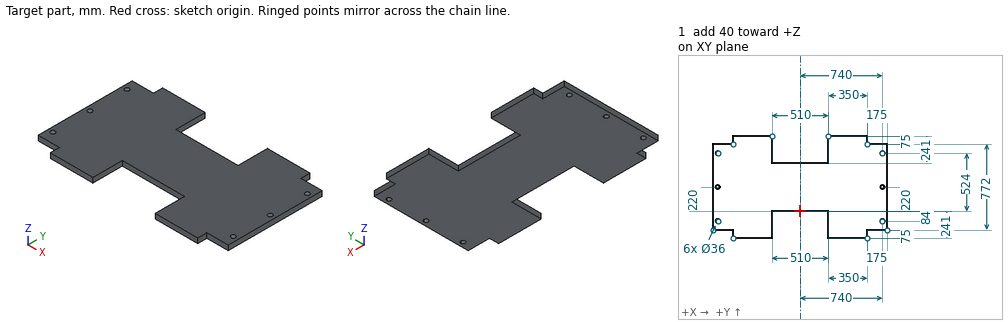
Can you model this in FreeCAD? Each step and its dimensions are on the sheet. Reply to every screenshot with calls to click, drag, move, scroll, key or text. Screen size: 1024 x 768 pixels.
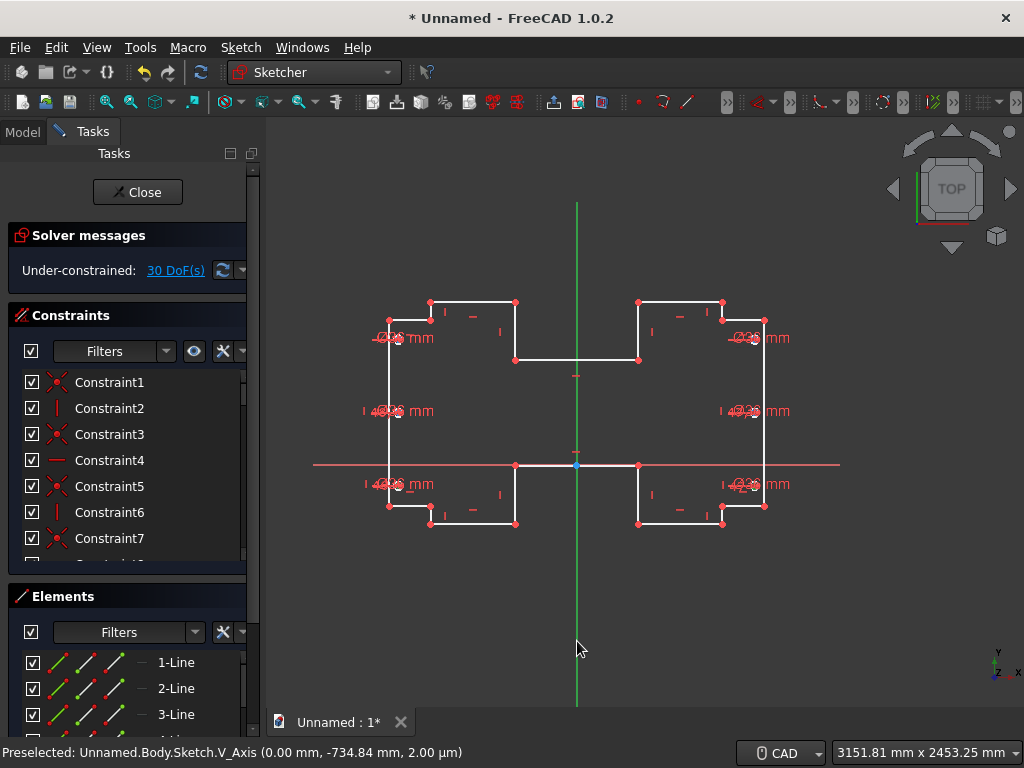
key(s)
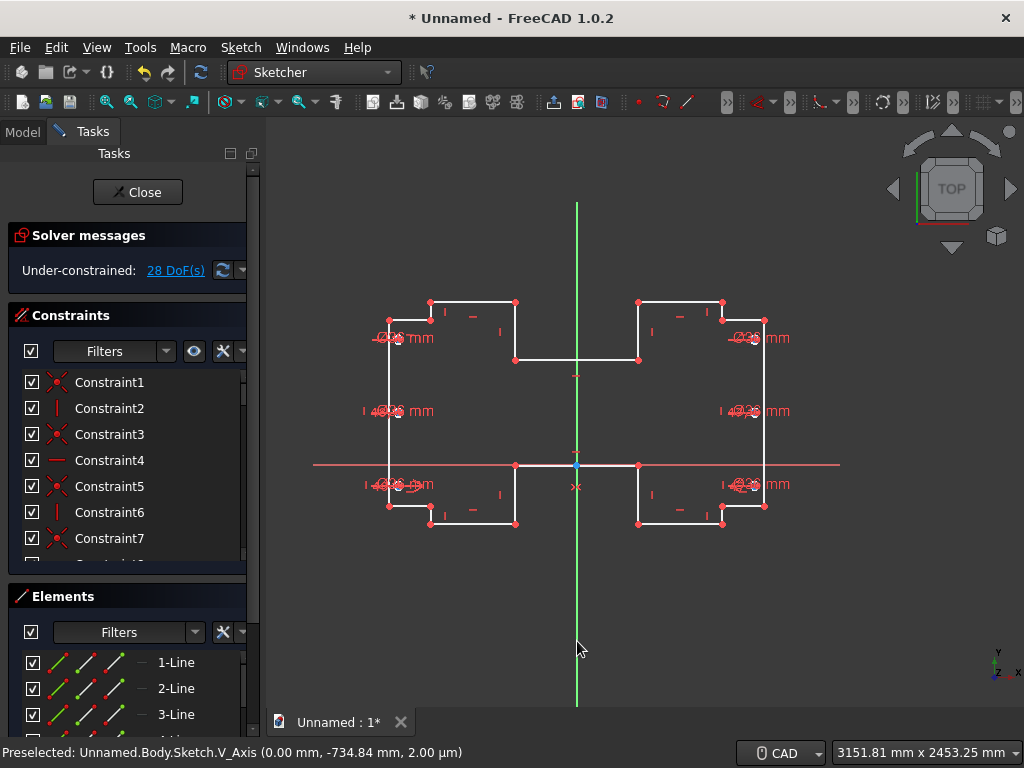
click(755, 340)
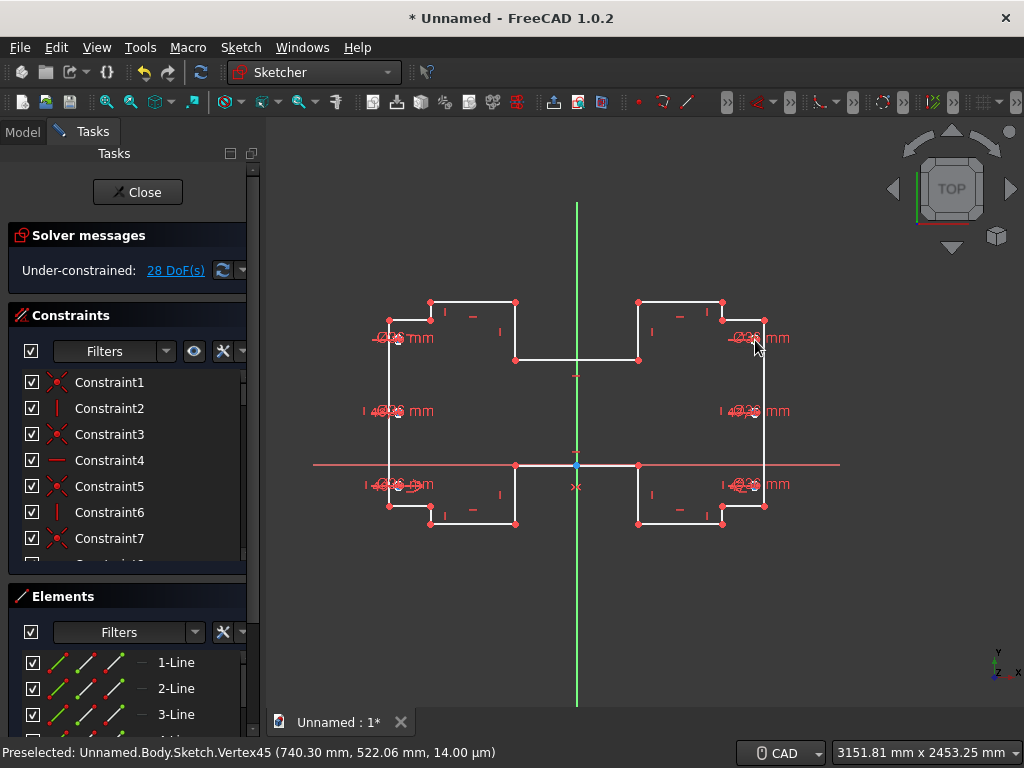
click(399, 340)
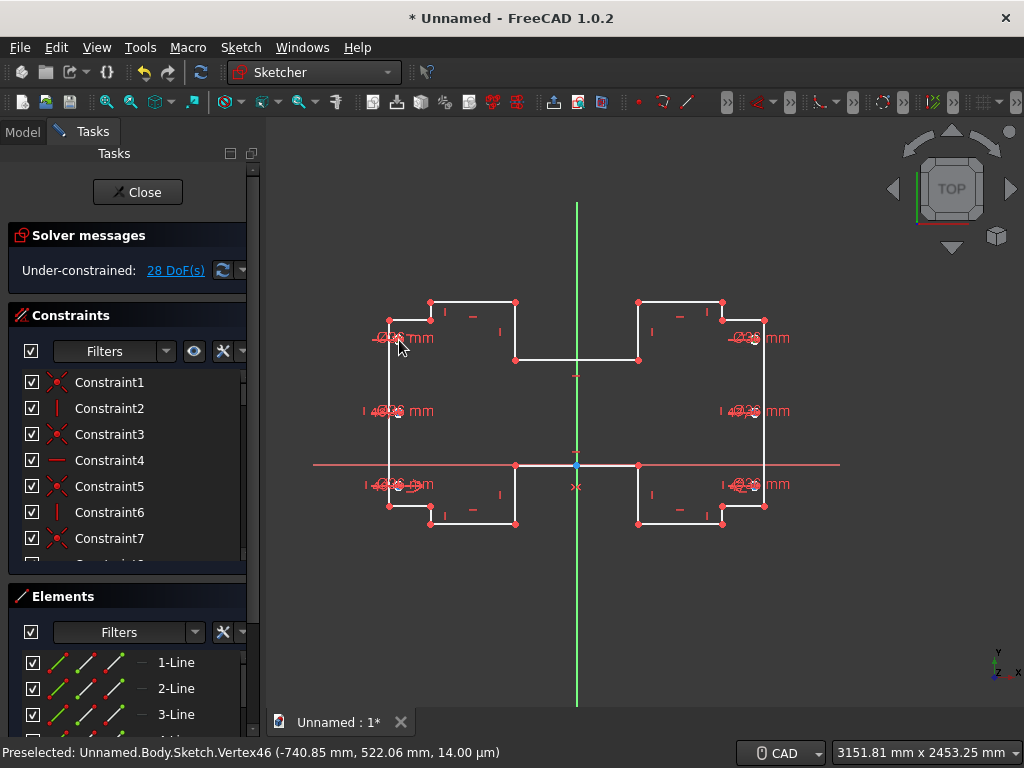
click(577, 641)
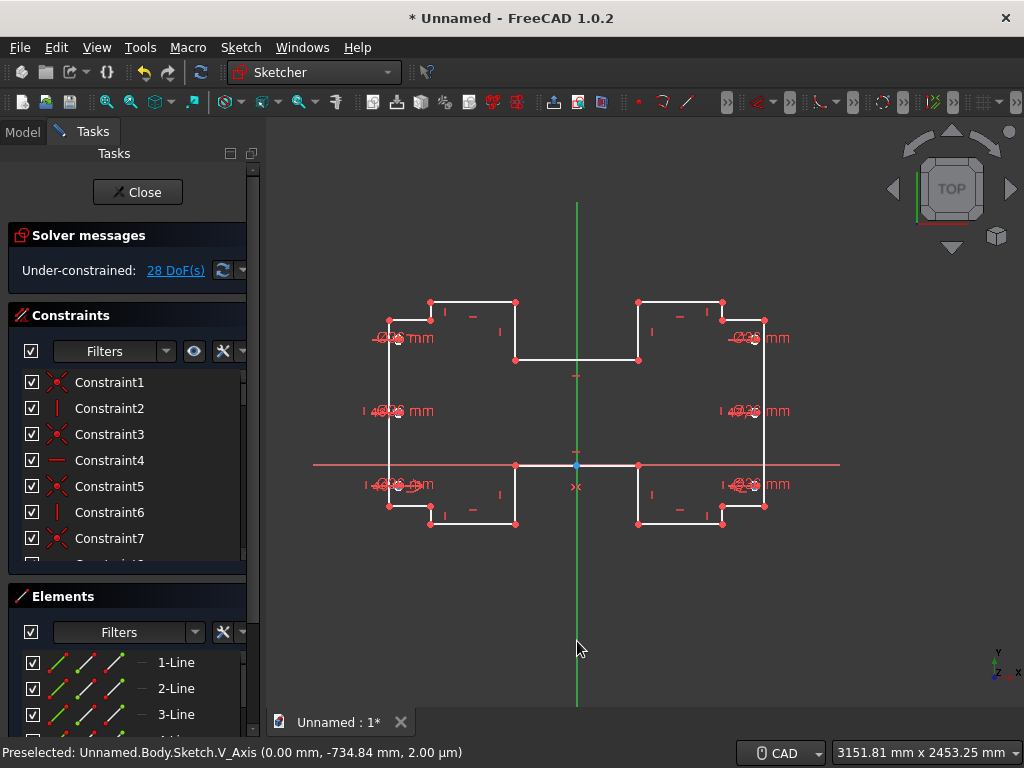
key(s)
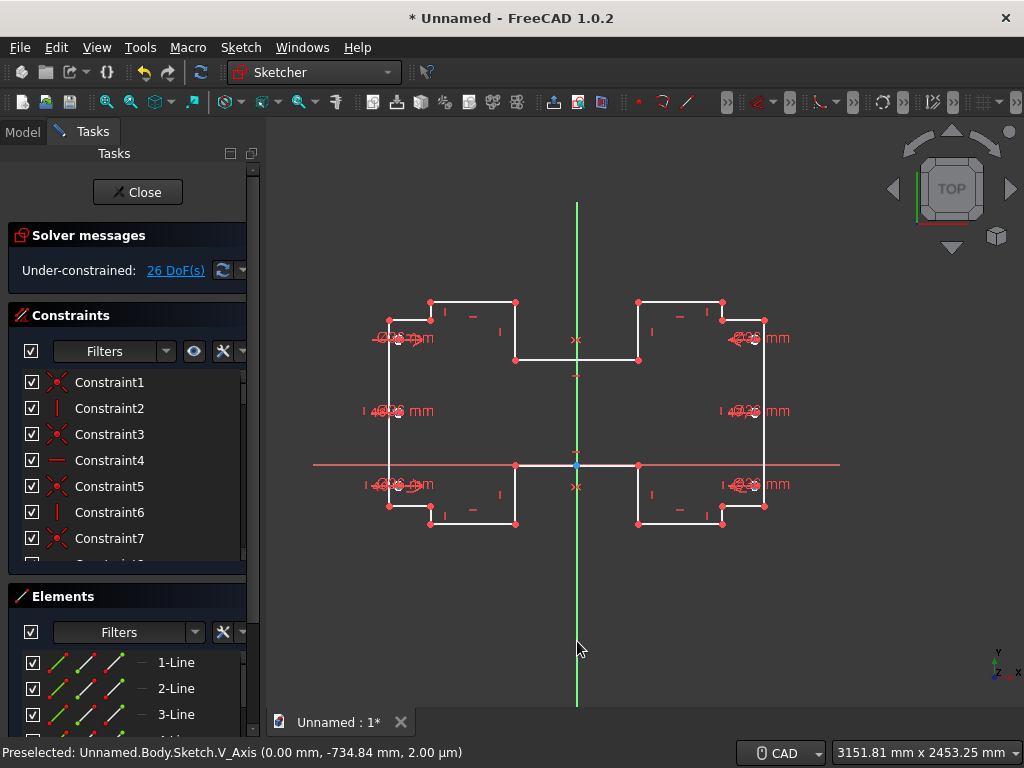
click(638, 302)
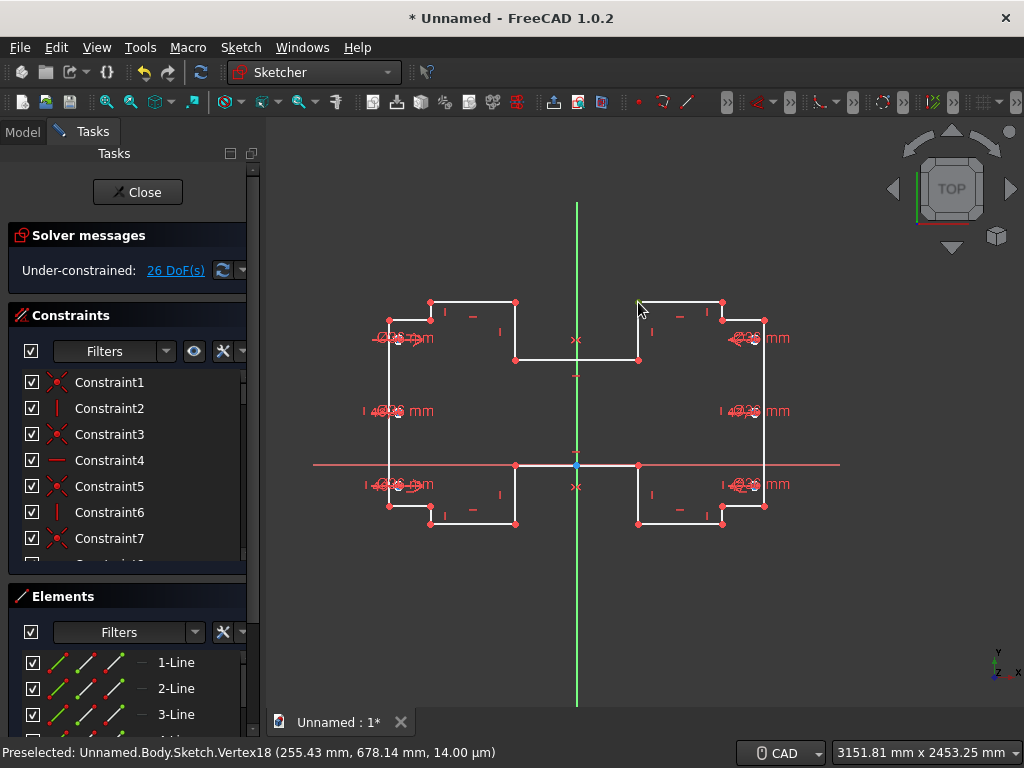
click(515, 302)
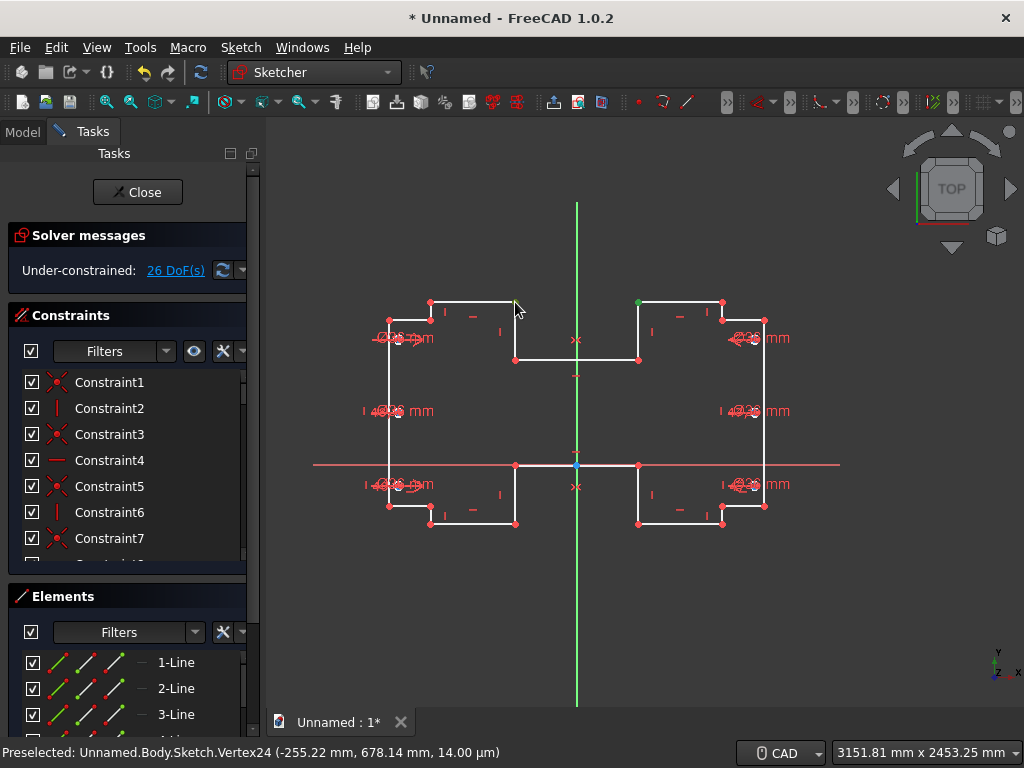
click(577, 641)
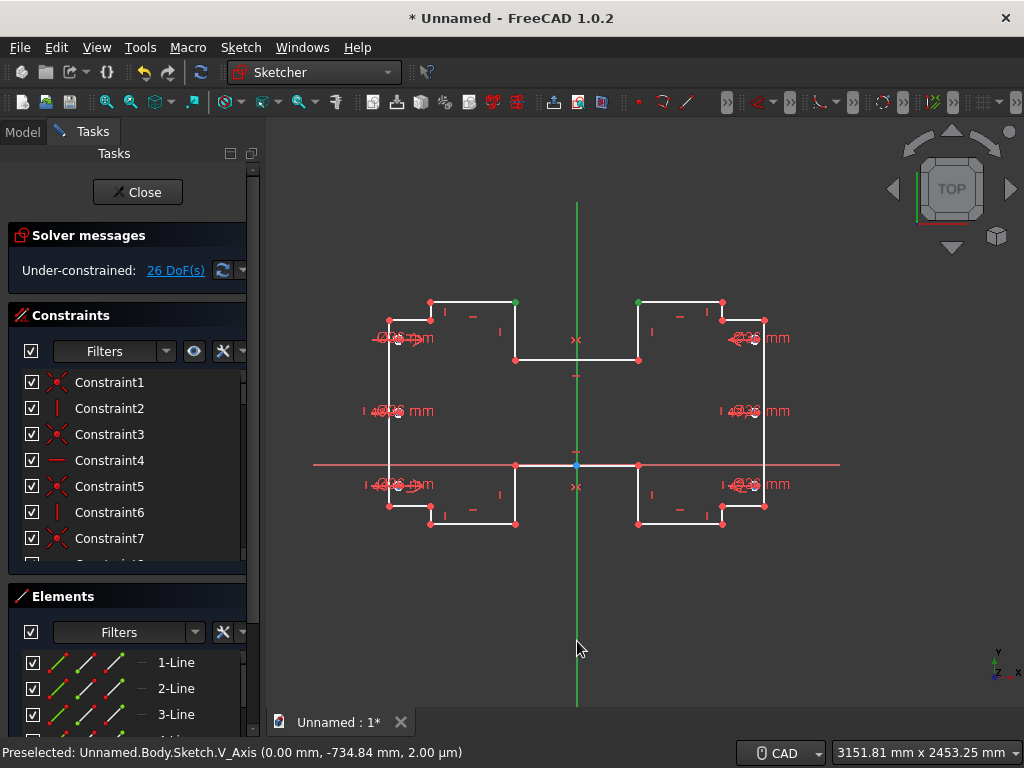
key(s)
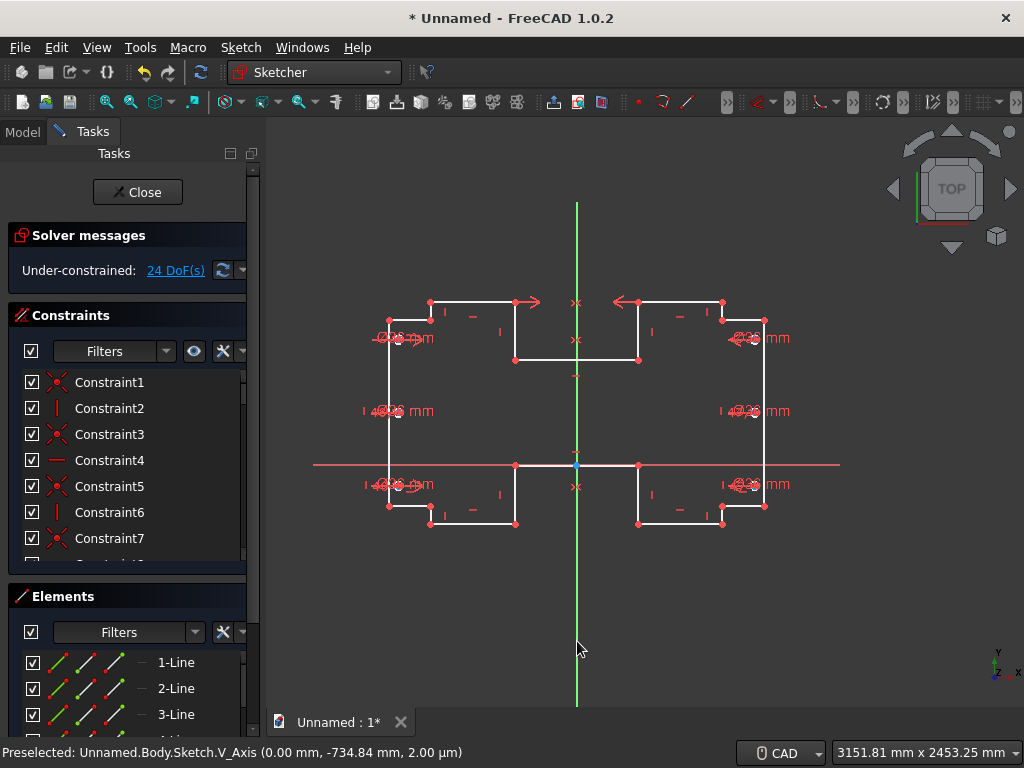
click(722, 320)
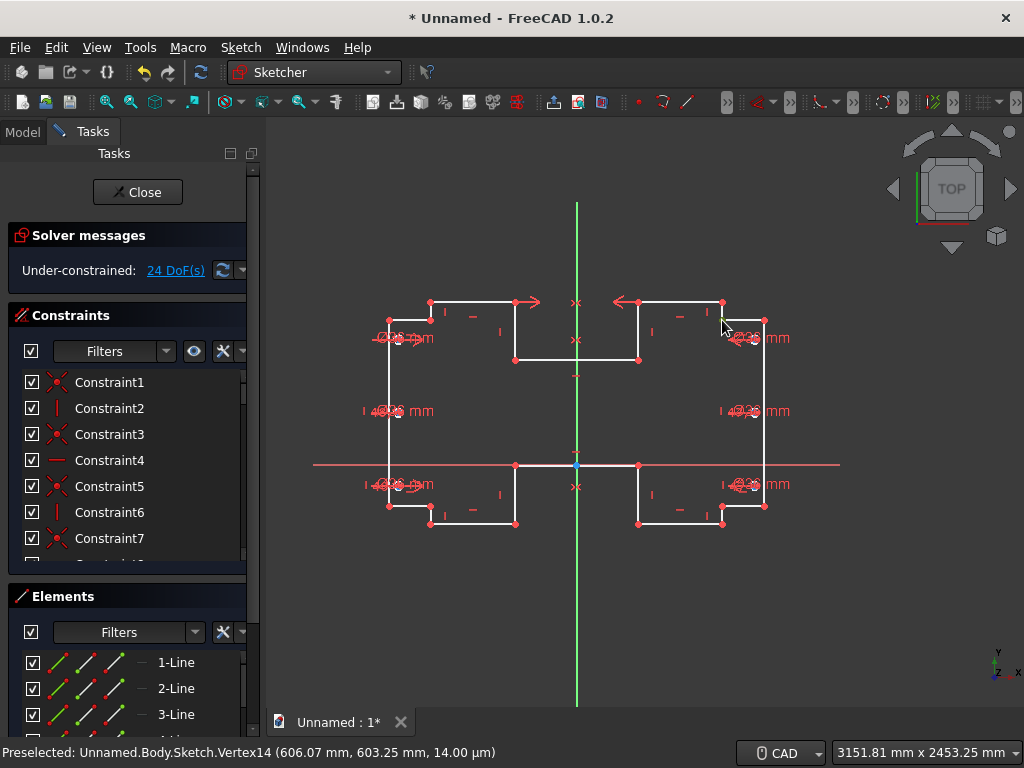
click(431, 320)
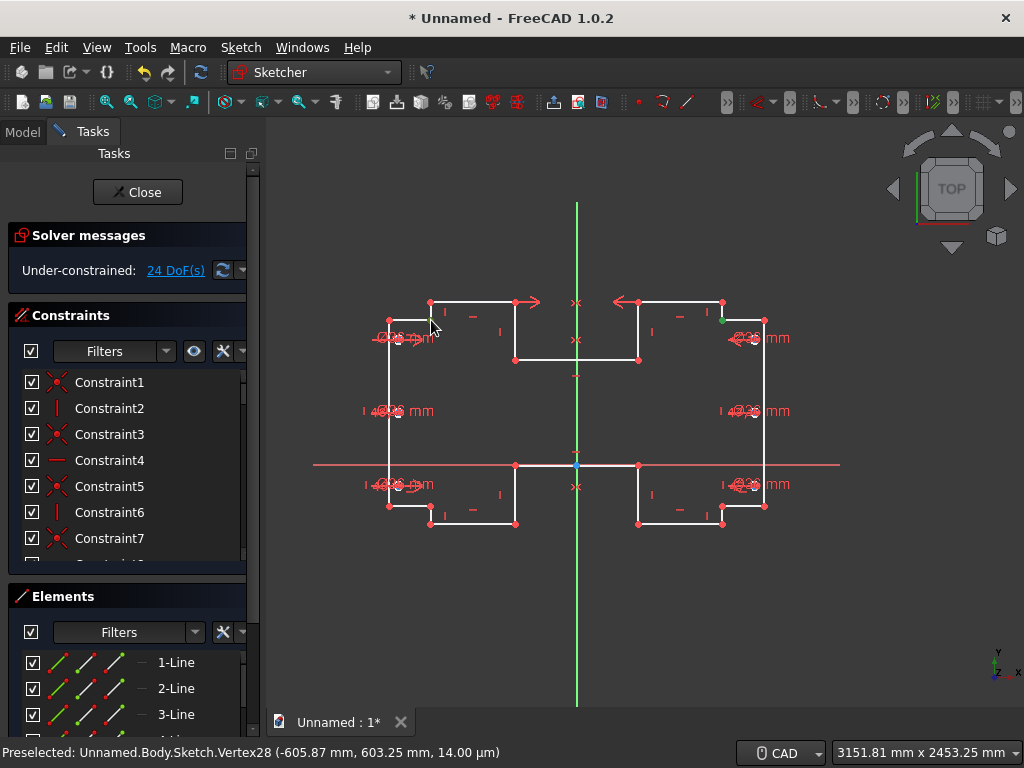
click(577, 641)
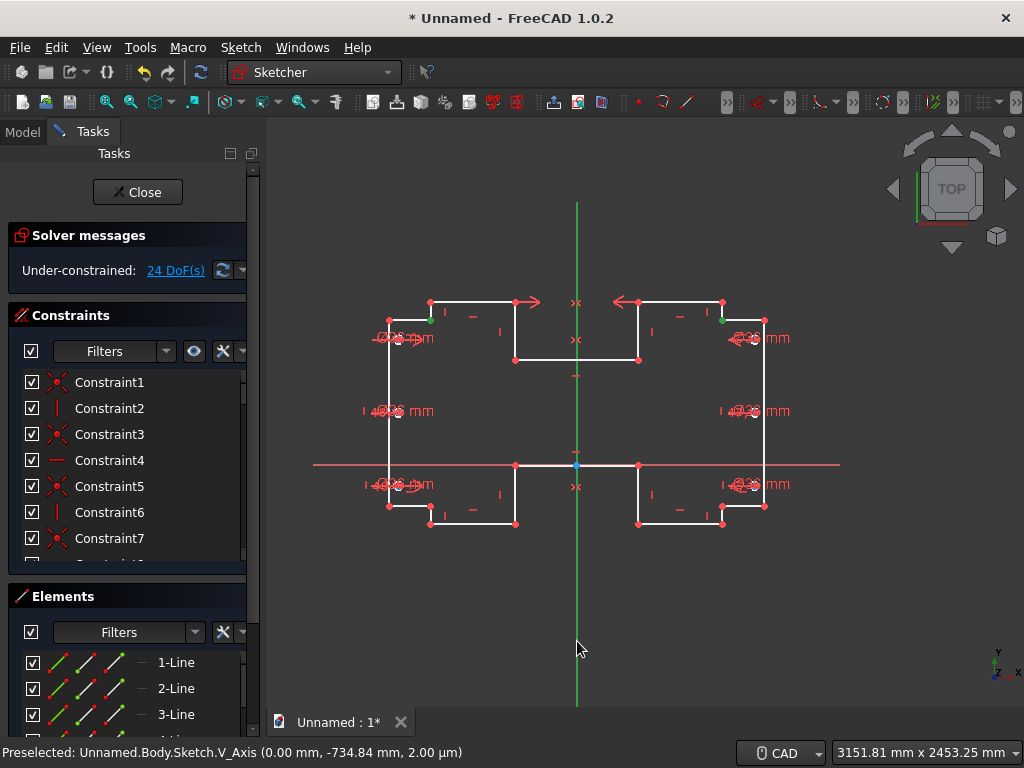
key(s)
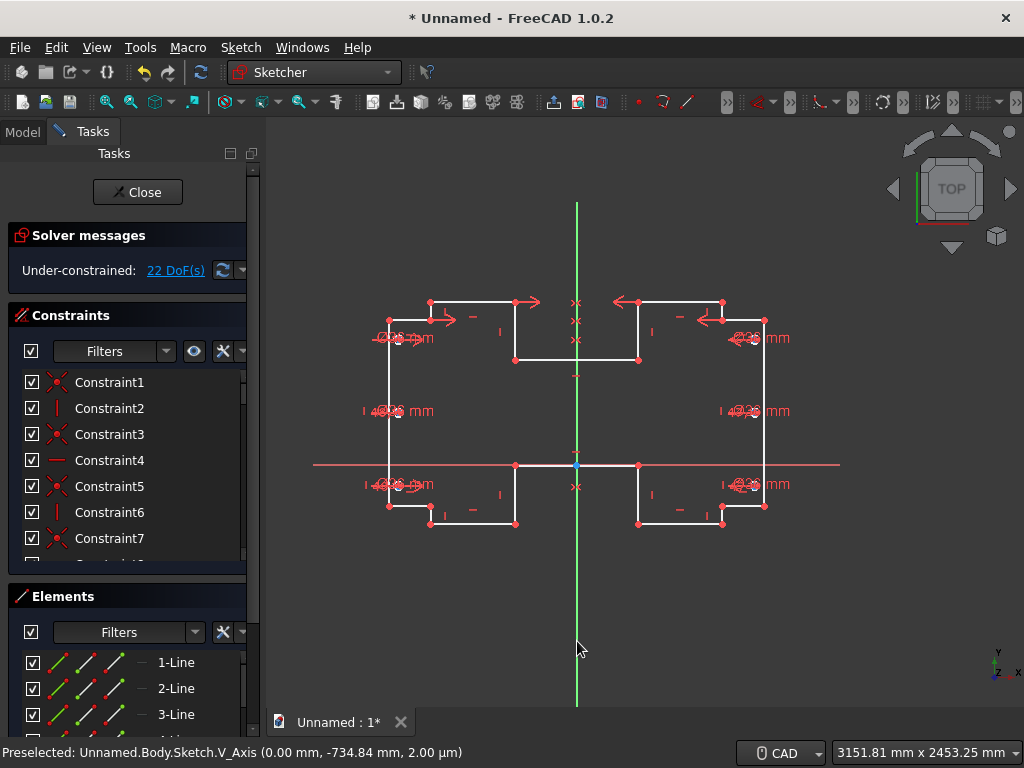
click(764, 506)